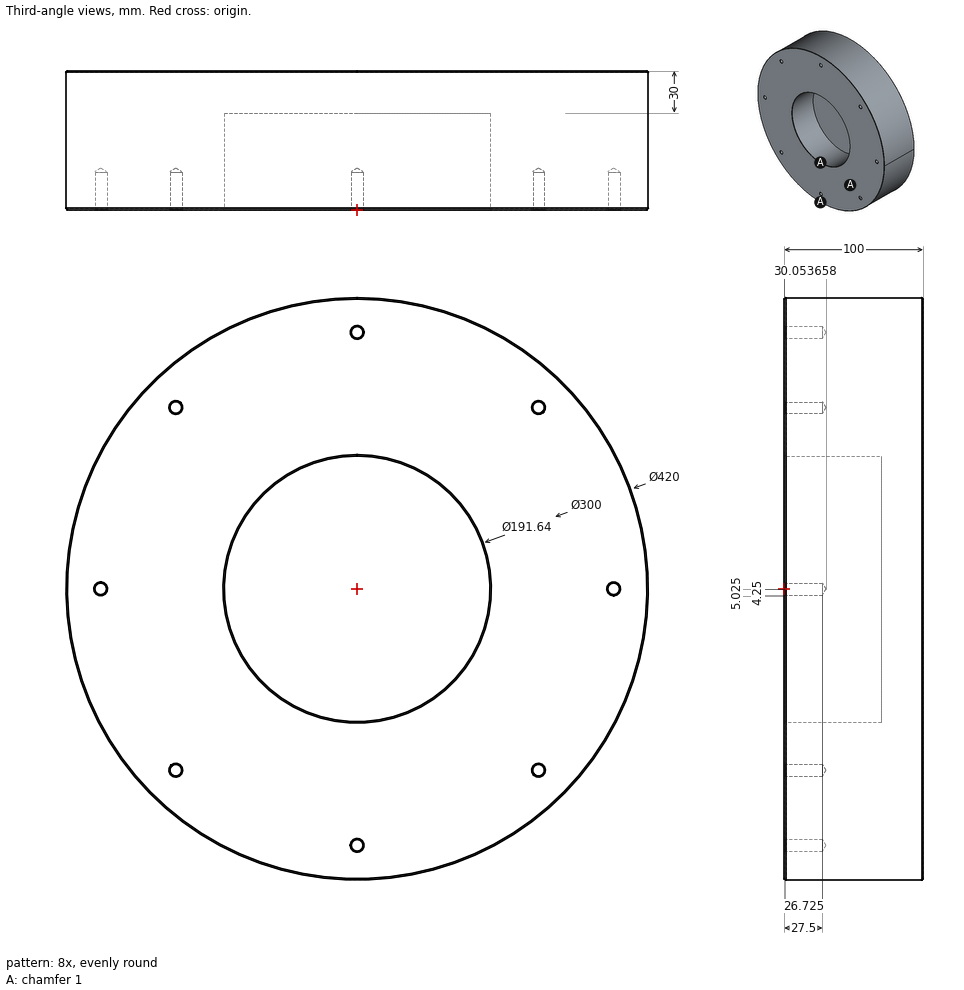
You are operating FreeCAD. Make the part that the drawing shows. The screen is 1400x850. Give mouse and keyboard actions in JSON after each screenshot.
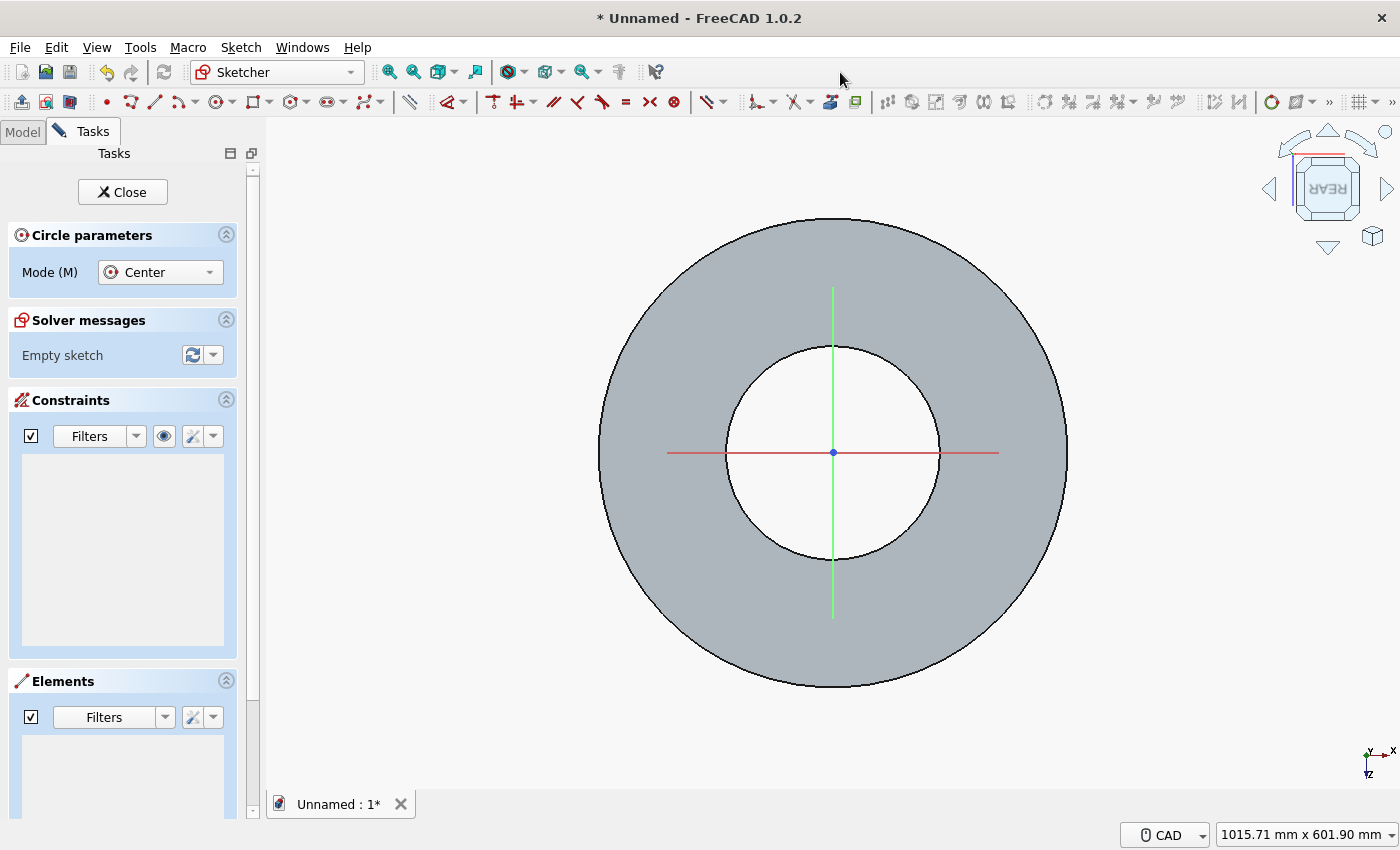
{"action": "left_click", "coordinate": [833, 453]}
{"action": "left_click", "coordinate": [951, 335]}
{"action": "key", "text": "Escape"}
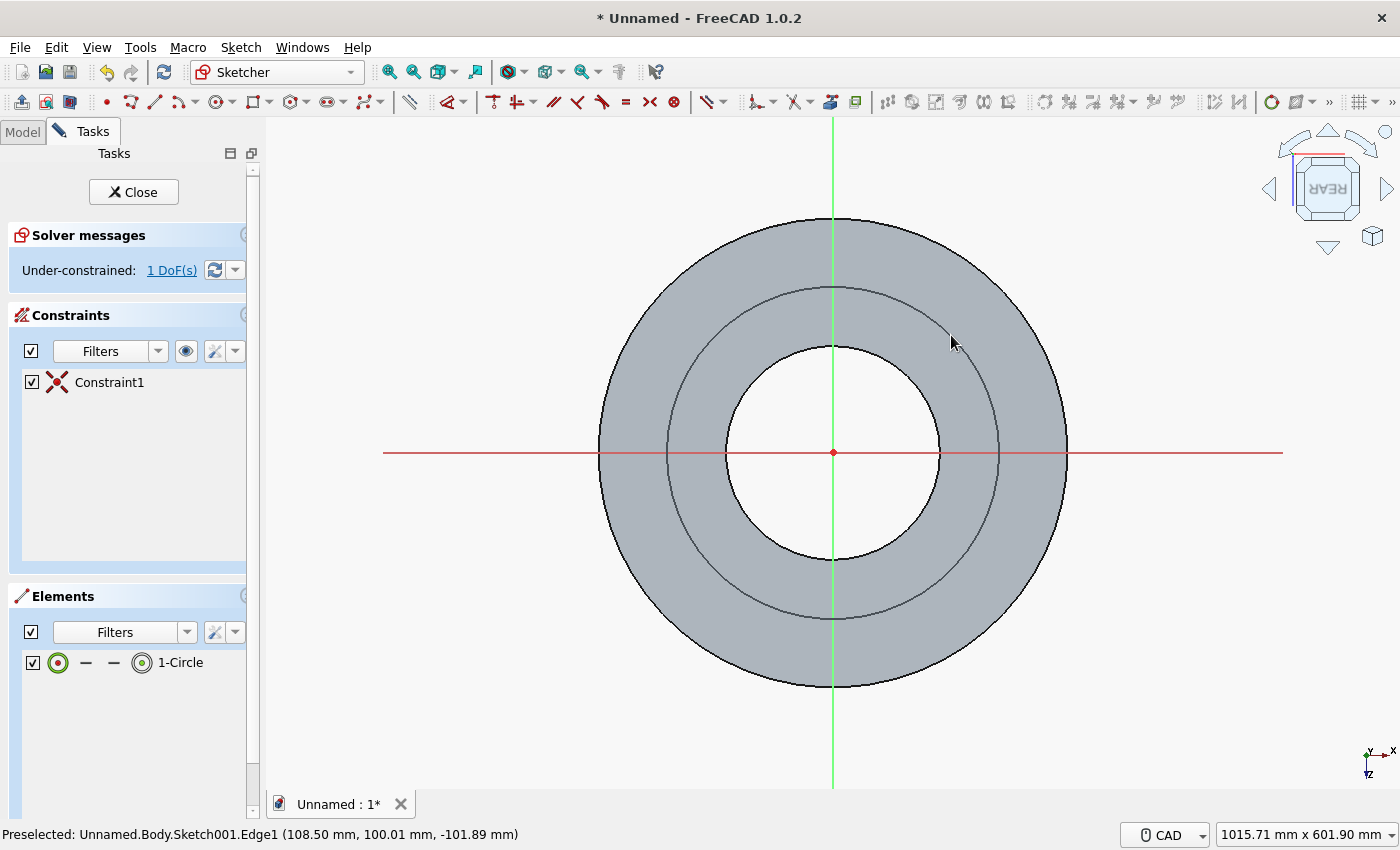
{"action": "left_click", "coordinate": [950, 335]}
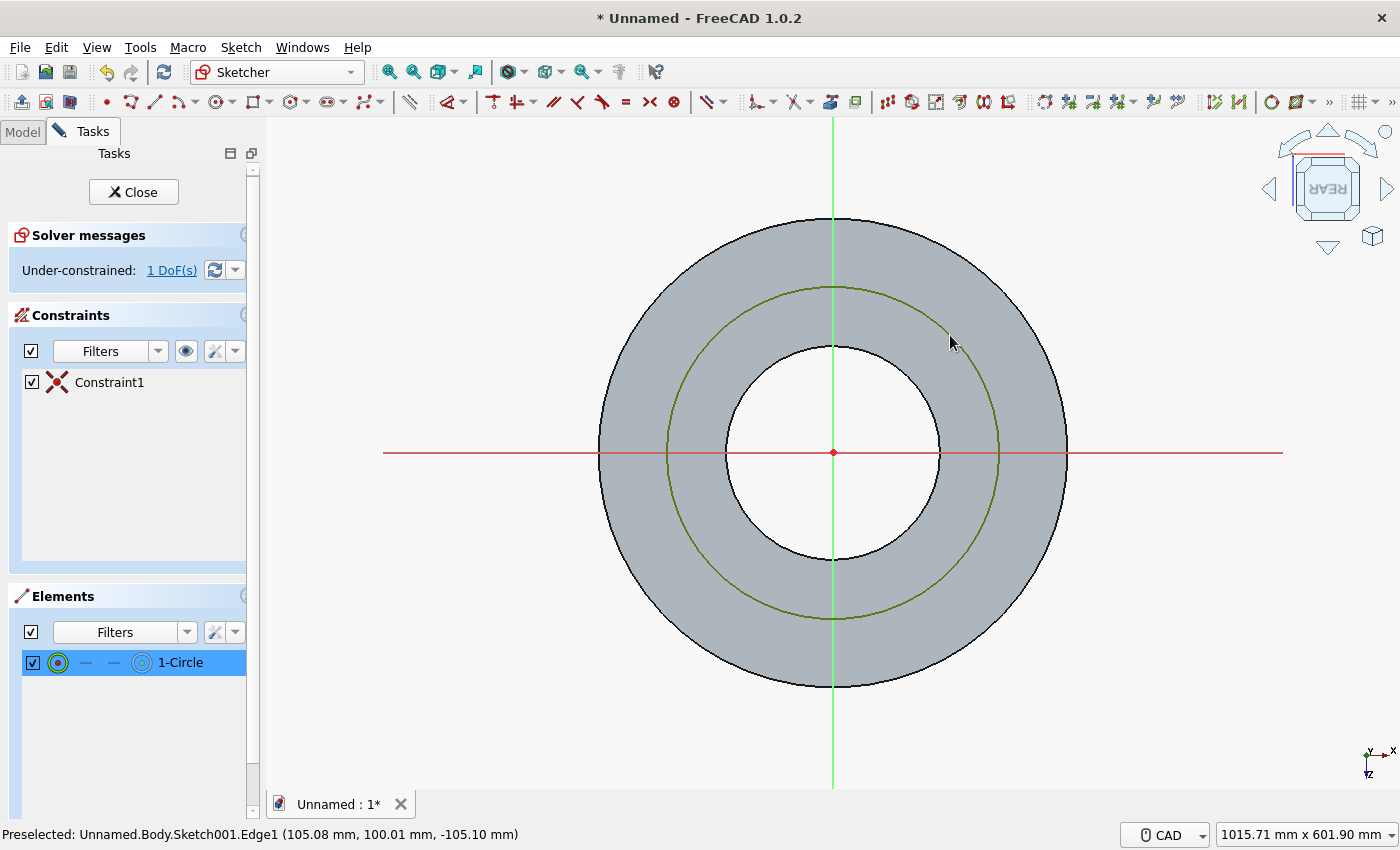
{"action": "key", "text": "k o"}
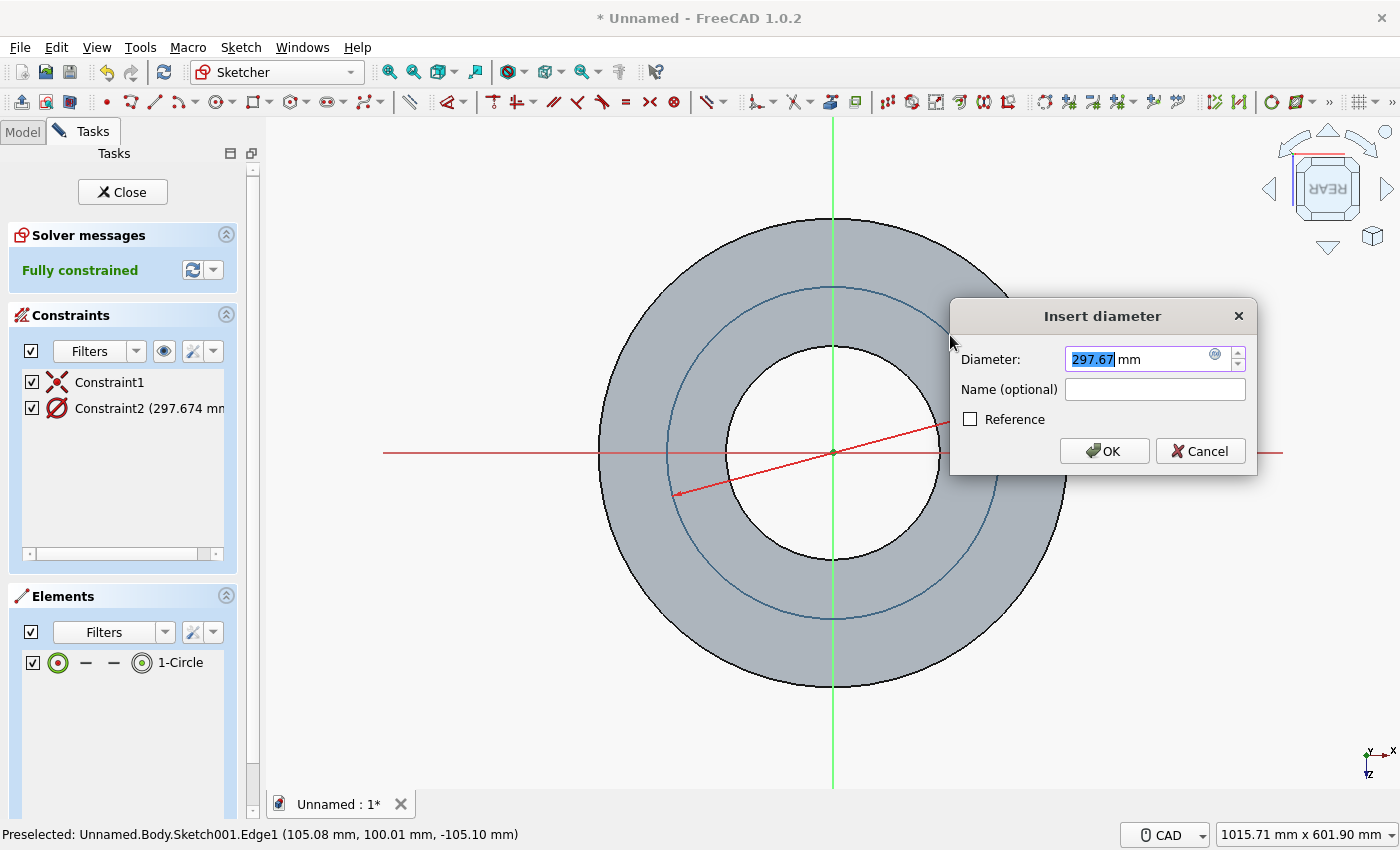
{"action": "type", "text": "300"}
{"action": "key", "text": "Return"}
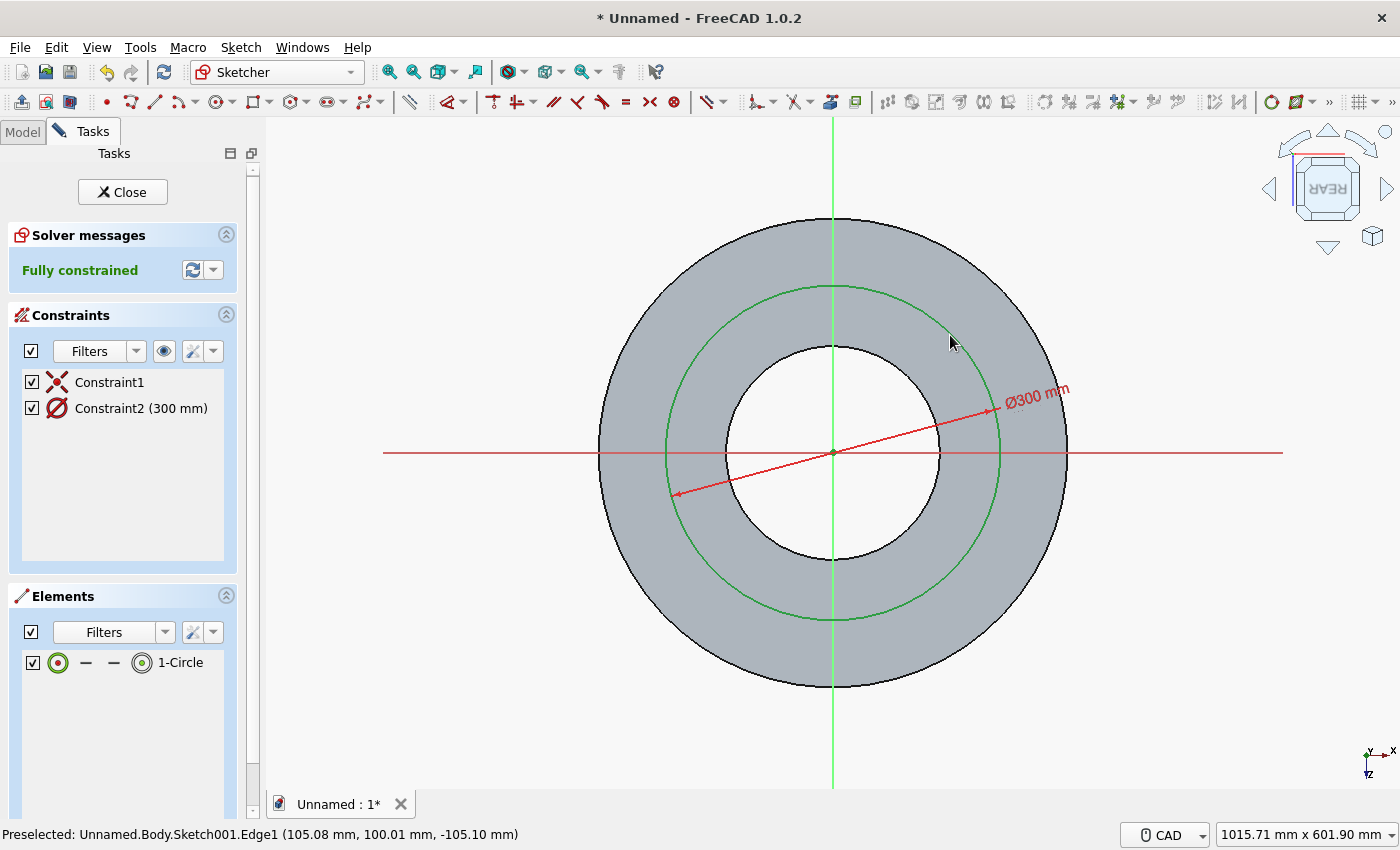
{"action": "left_click", "coordinate": [123, 192]}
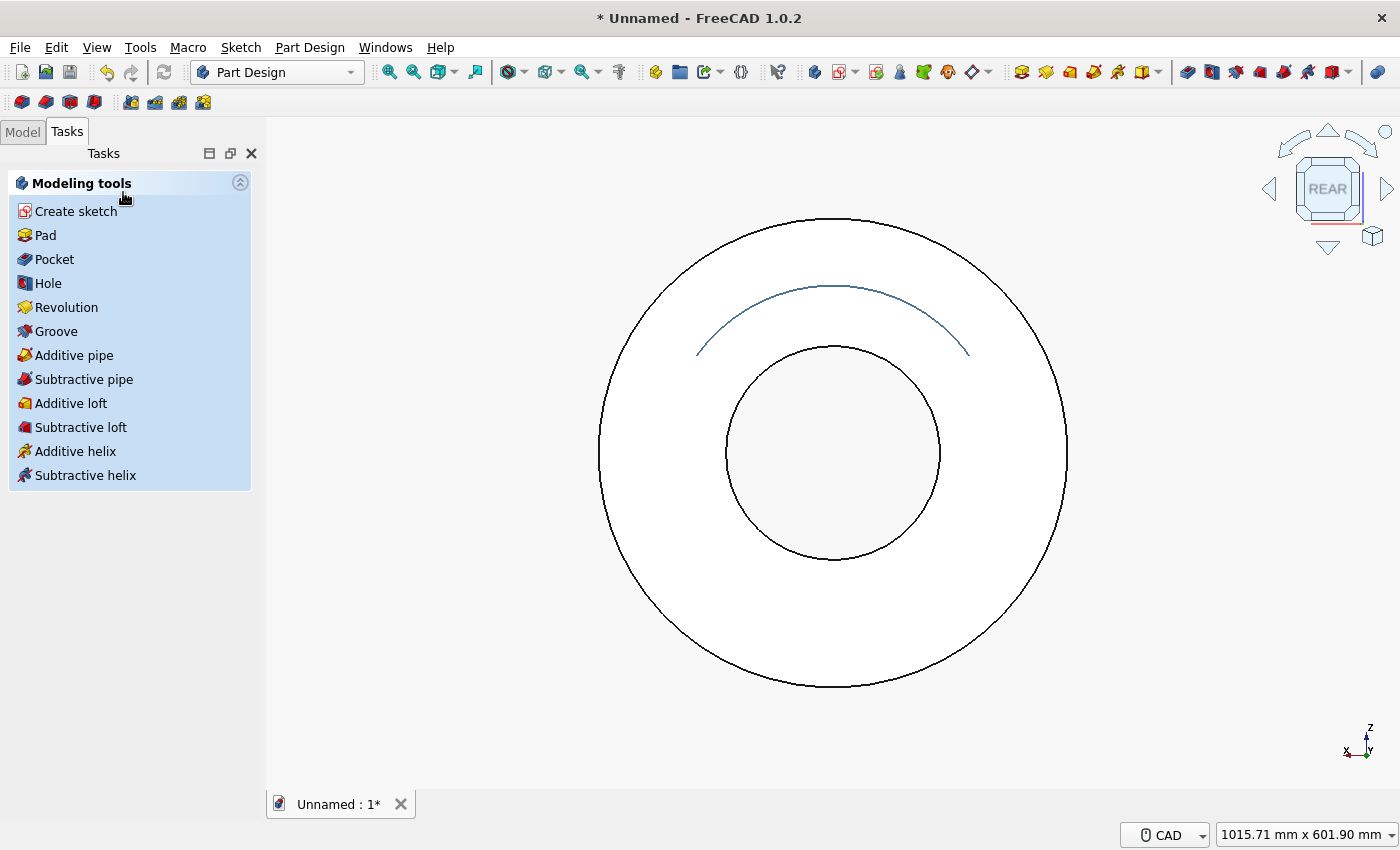
{"action": "left_click", "coordinate": [1022, 72]}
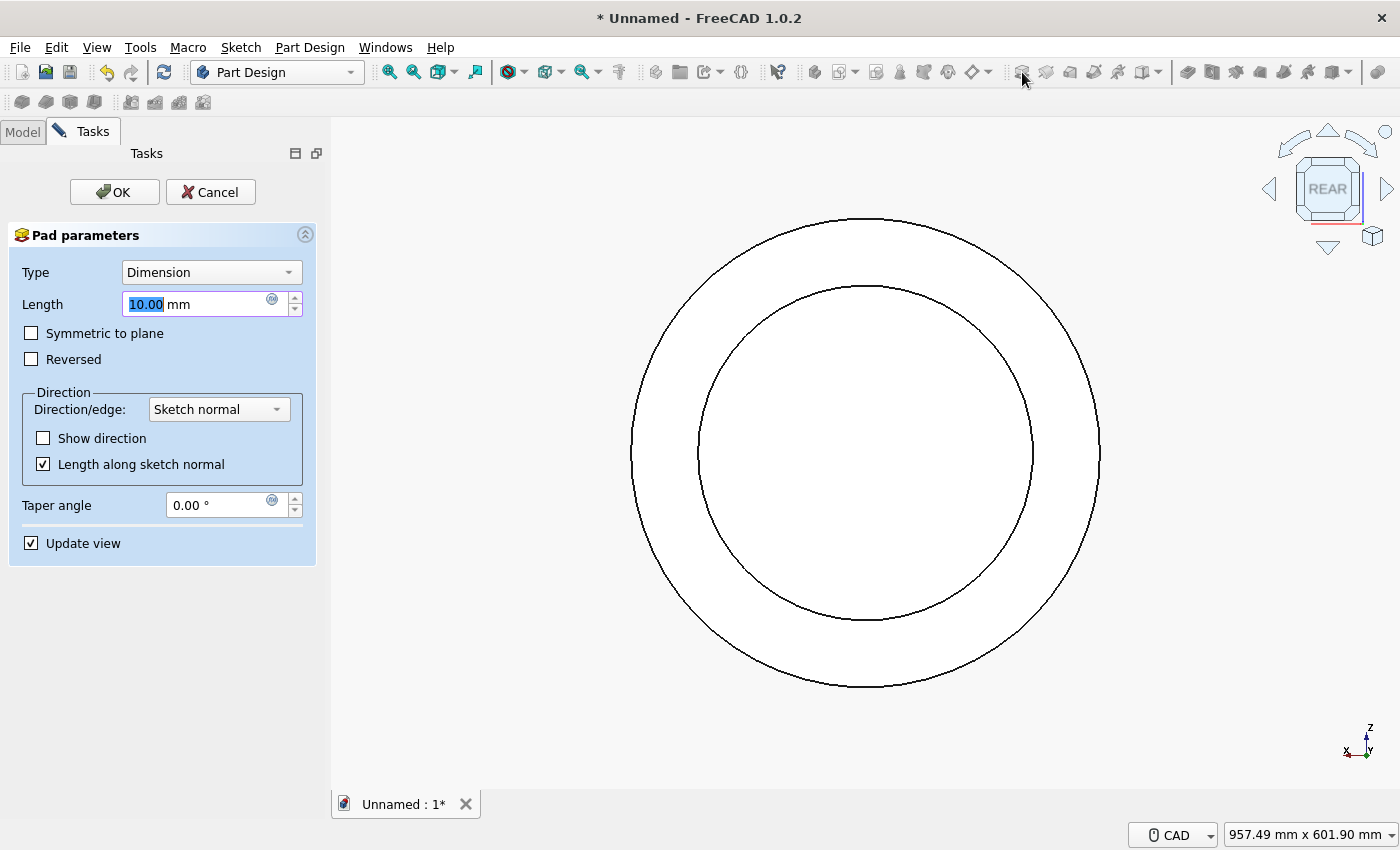
{"action": "type", "text": "30"}
{"action": "key", "text": "Tab"}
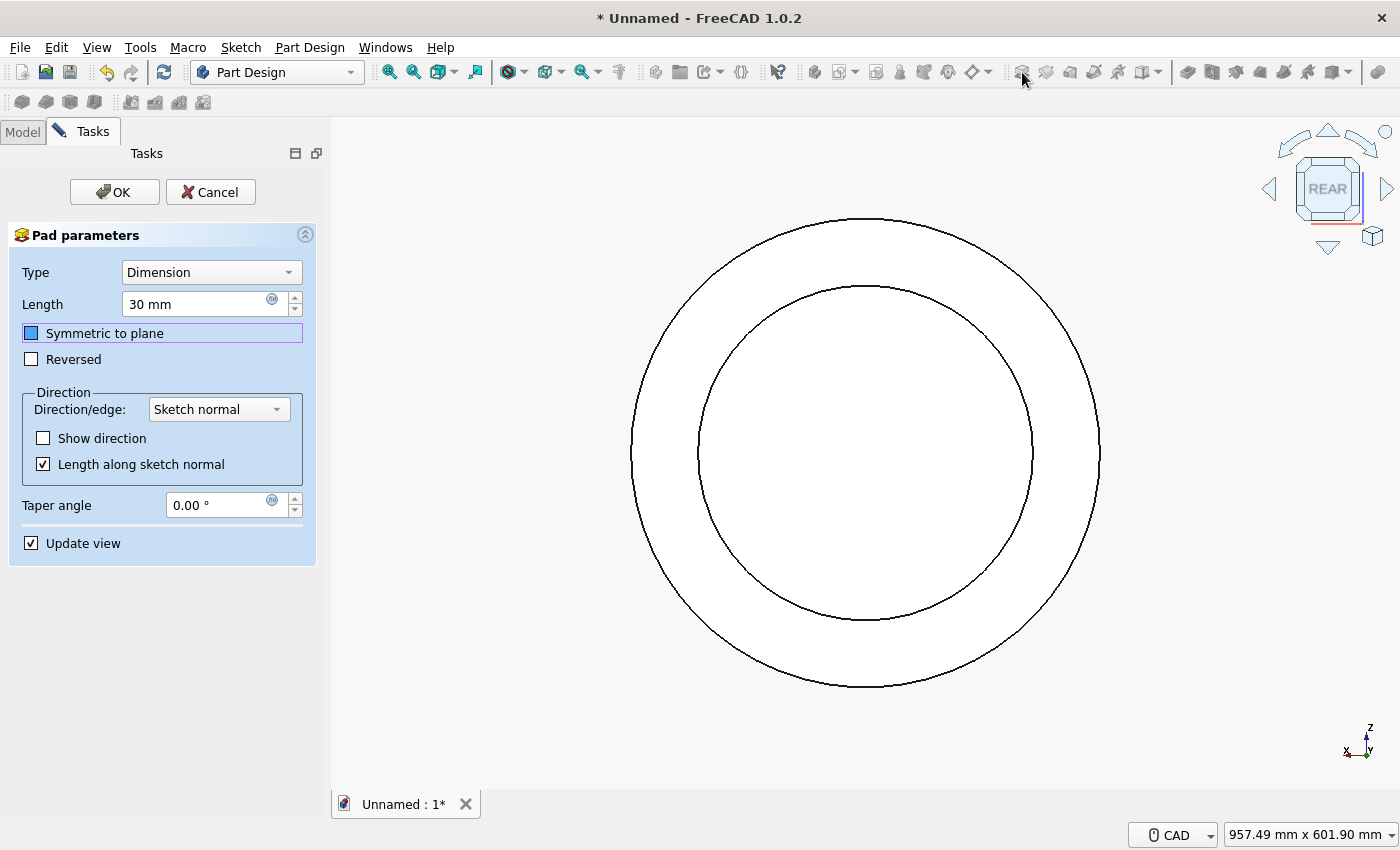
{"action": "left_click", "coordinate": [30, 359]}